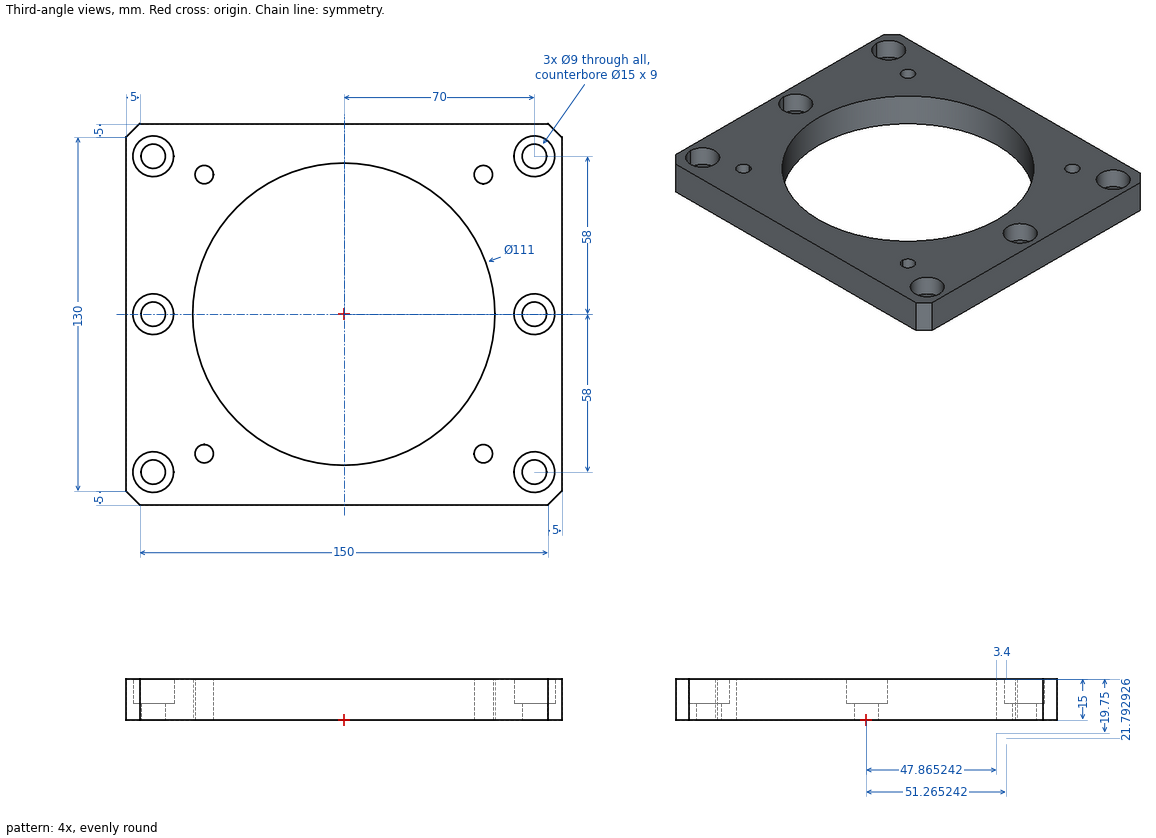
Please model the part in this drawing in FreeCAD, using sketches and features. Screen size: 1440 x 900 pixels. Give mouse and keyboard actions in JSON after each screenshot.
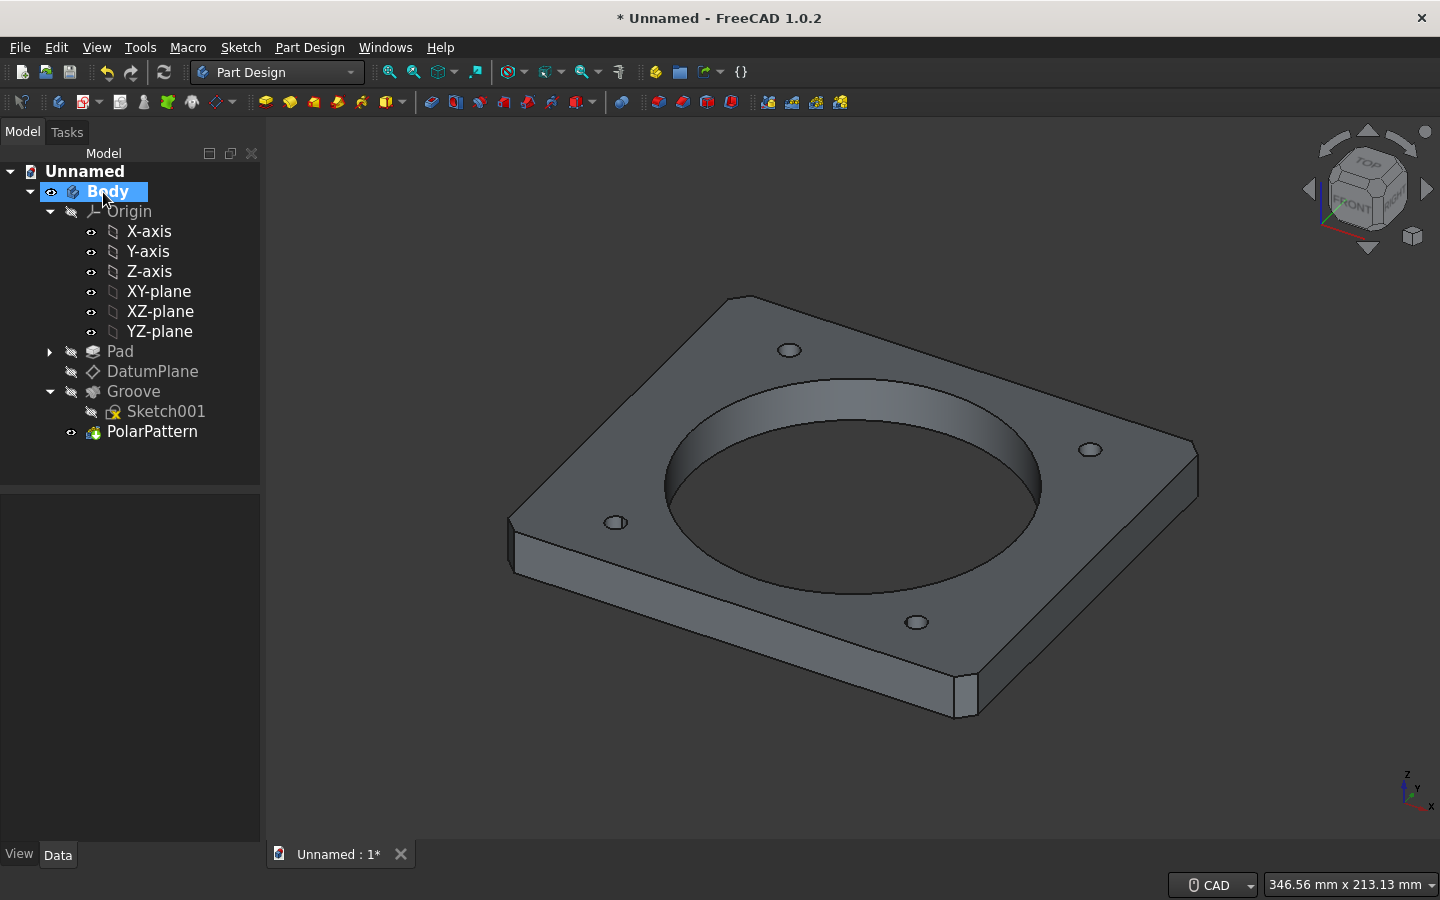
{"action": "left_click", "coordinate": [720, 351]}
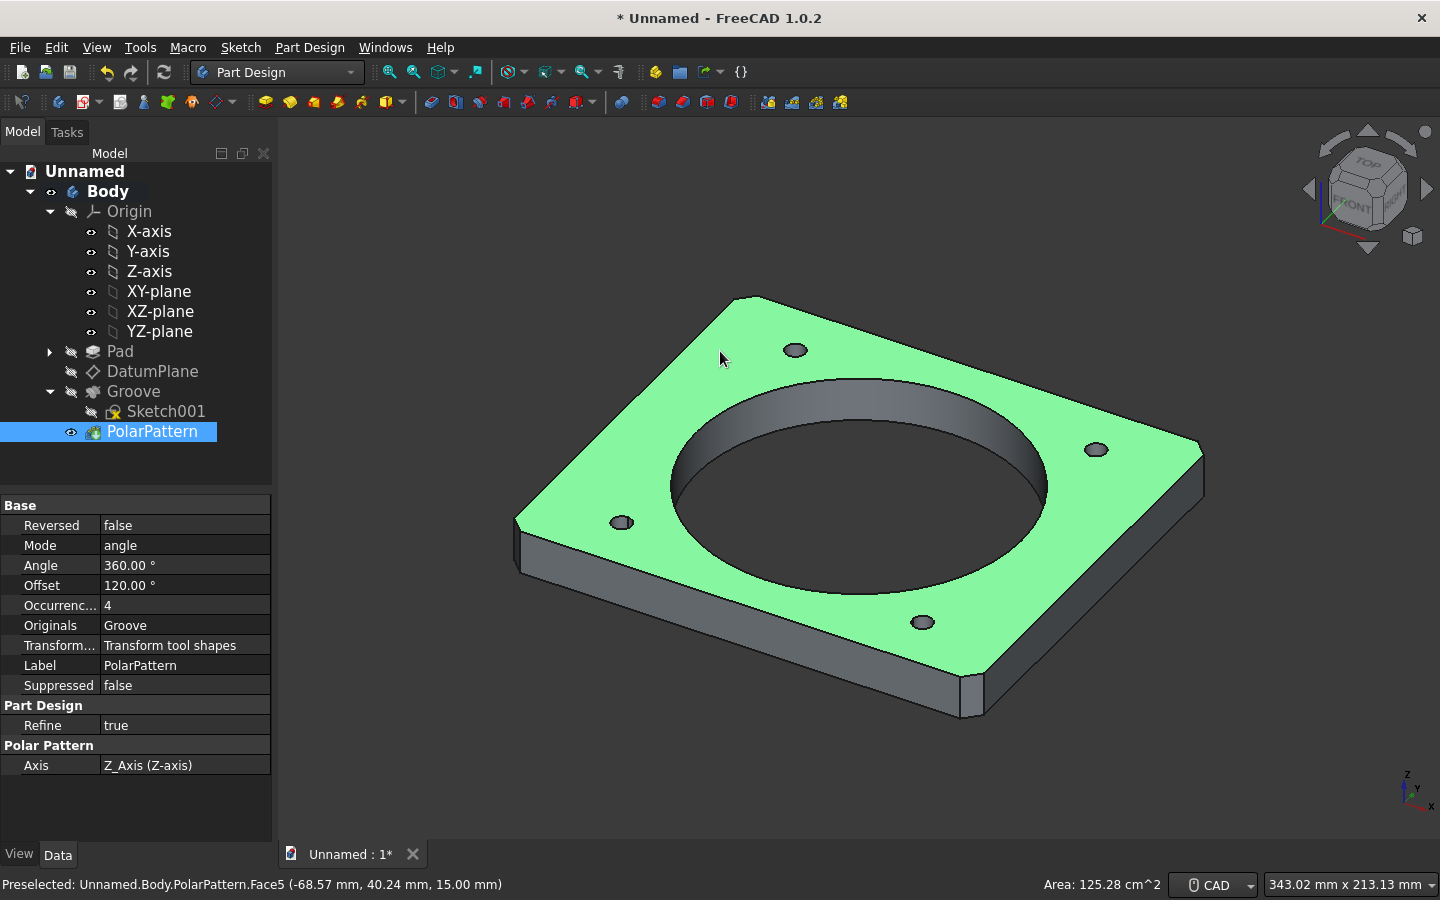
{"action": "left_click", "coordinate": [84, 102]}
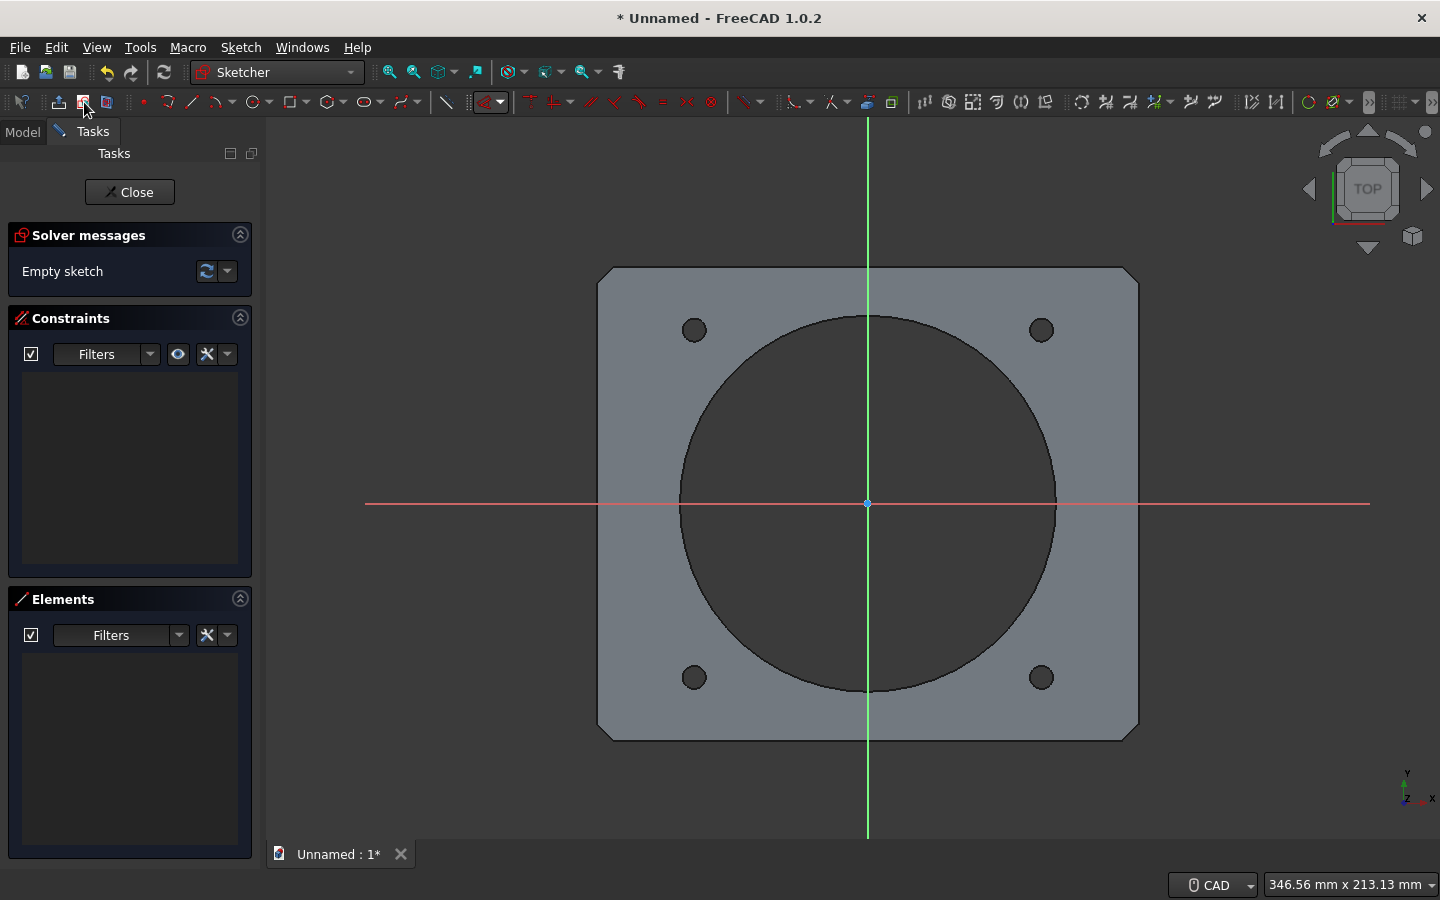
{"action": "left_click", "coordinate": [254, 102]}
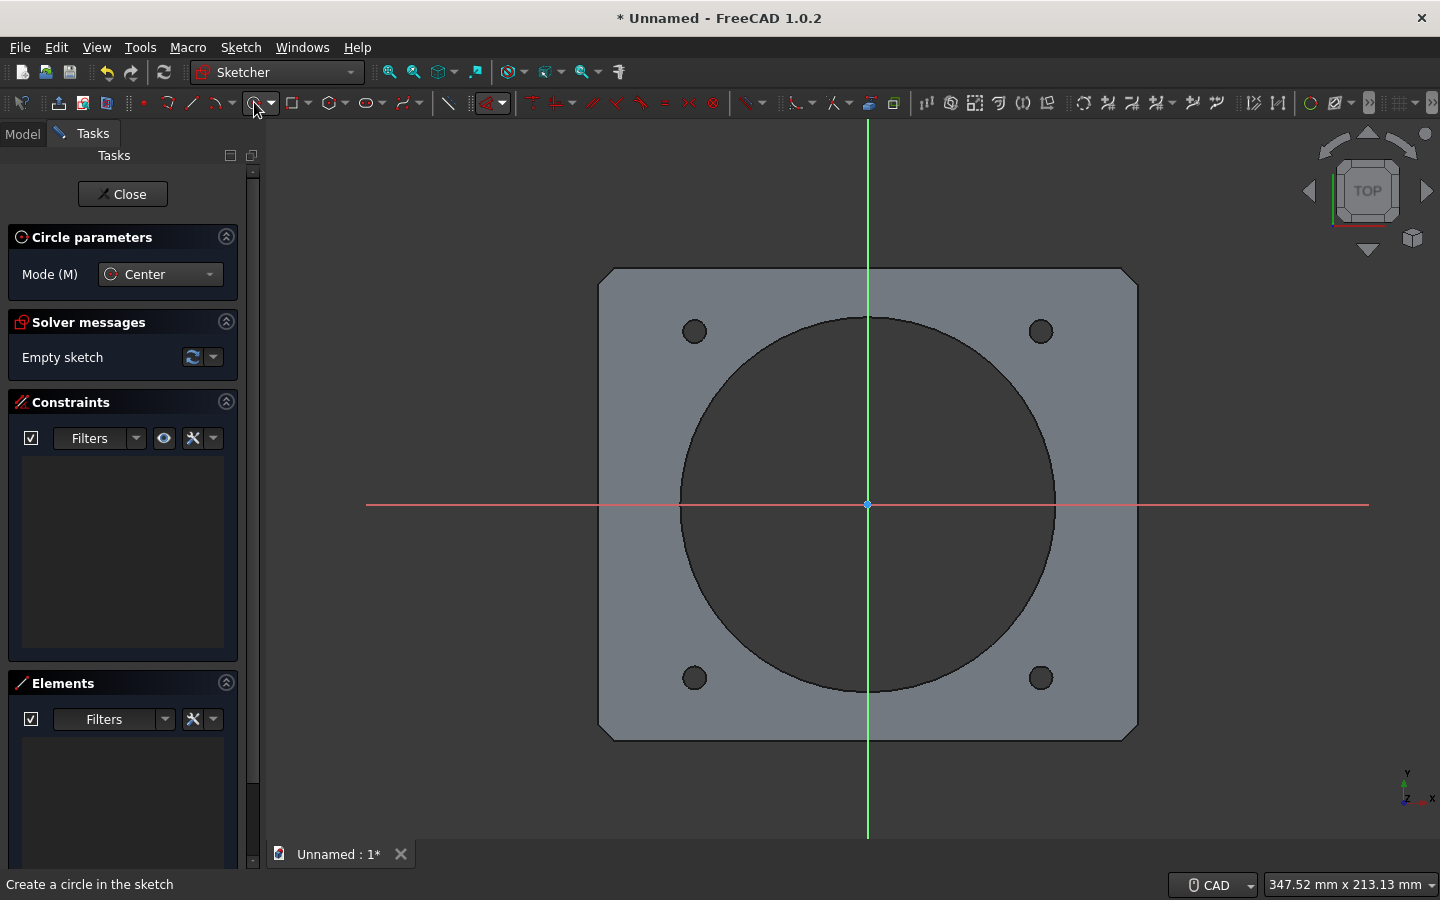
{"action": "scroll", "coordinate": [1104, 309], "scroll_direction": "up", "scroll_amount": 3}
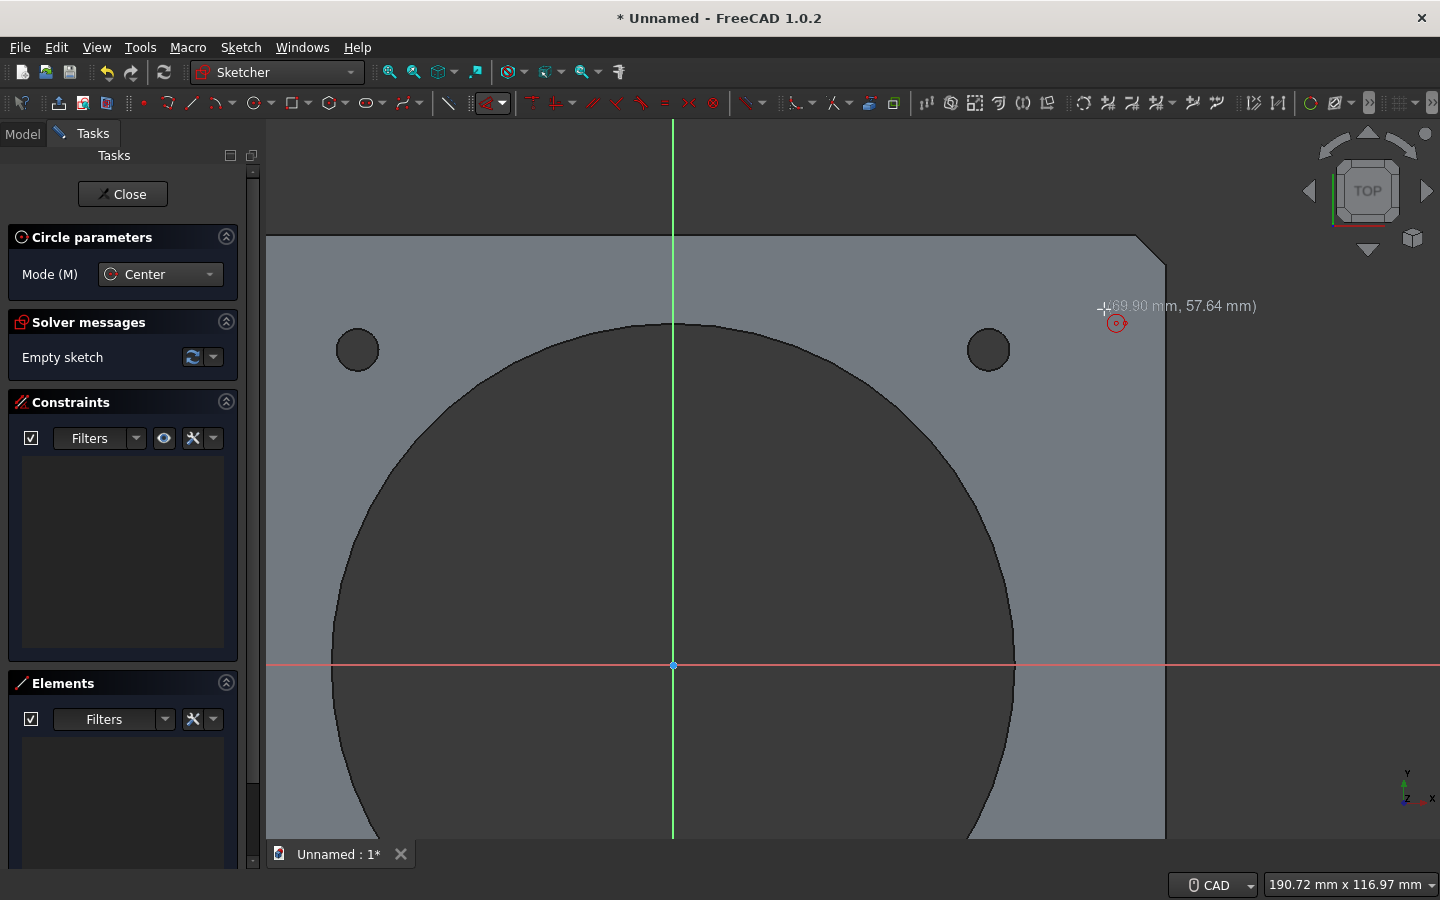
{"action": "left_click", "coordinate": [1104, 308]}
{"action": "mouse_move", "coordinate": [1124, 289]}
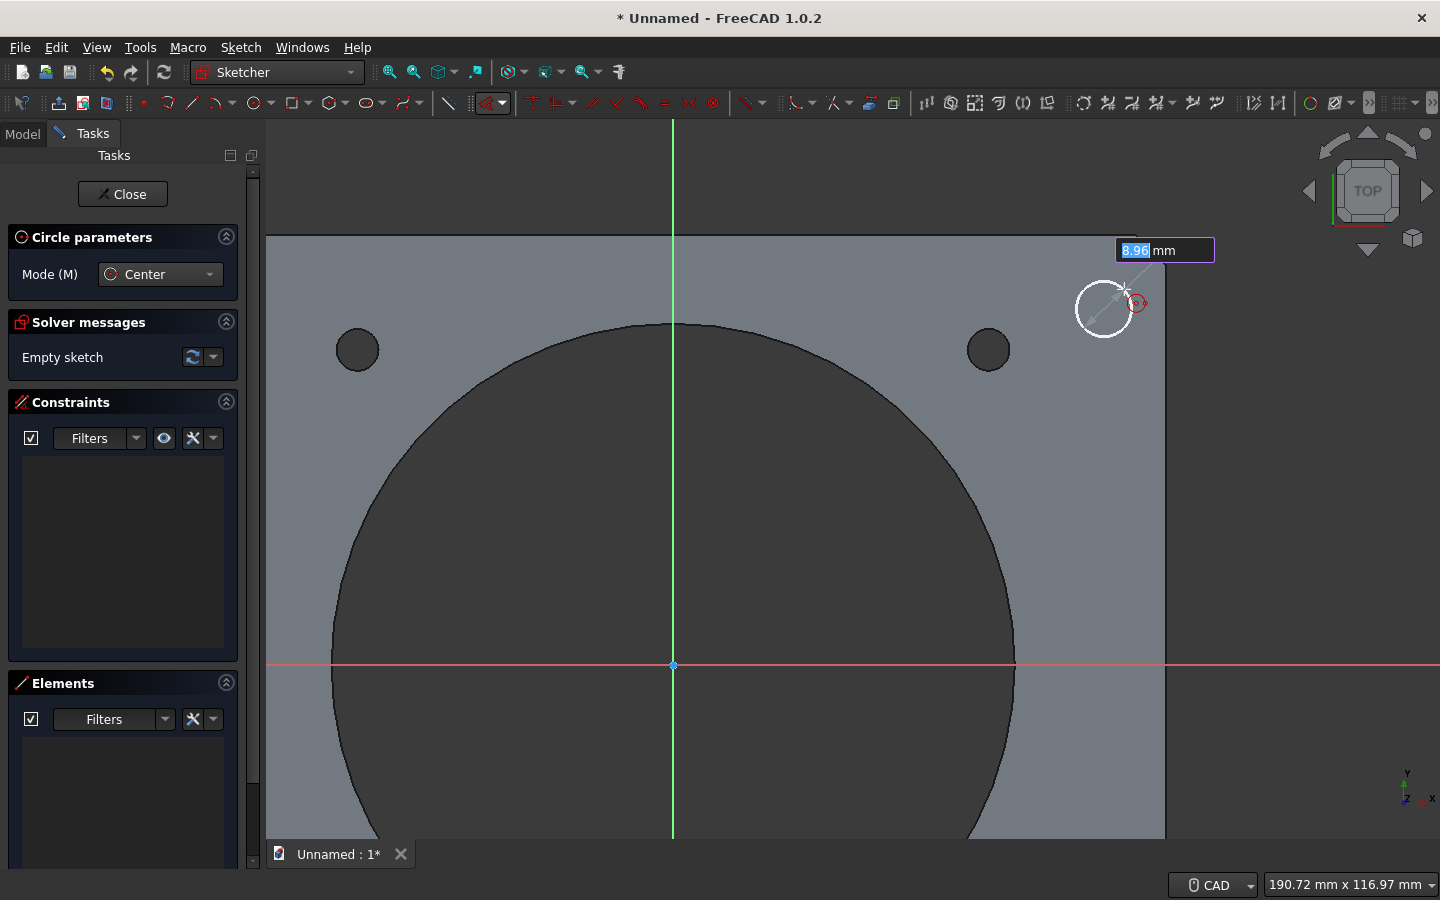
{"action": "type", "text": "9"}
{"action": "key", "text": "Return"}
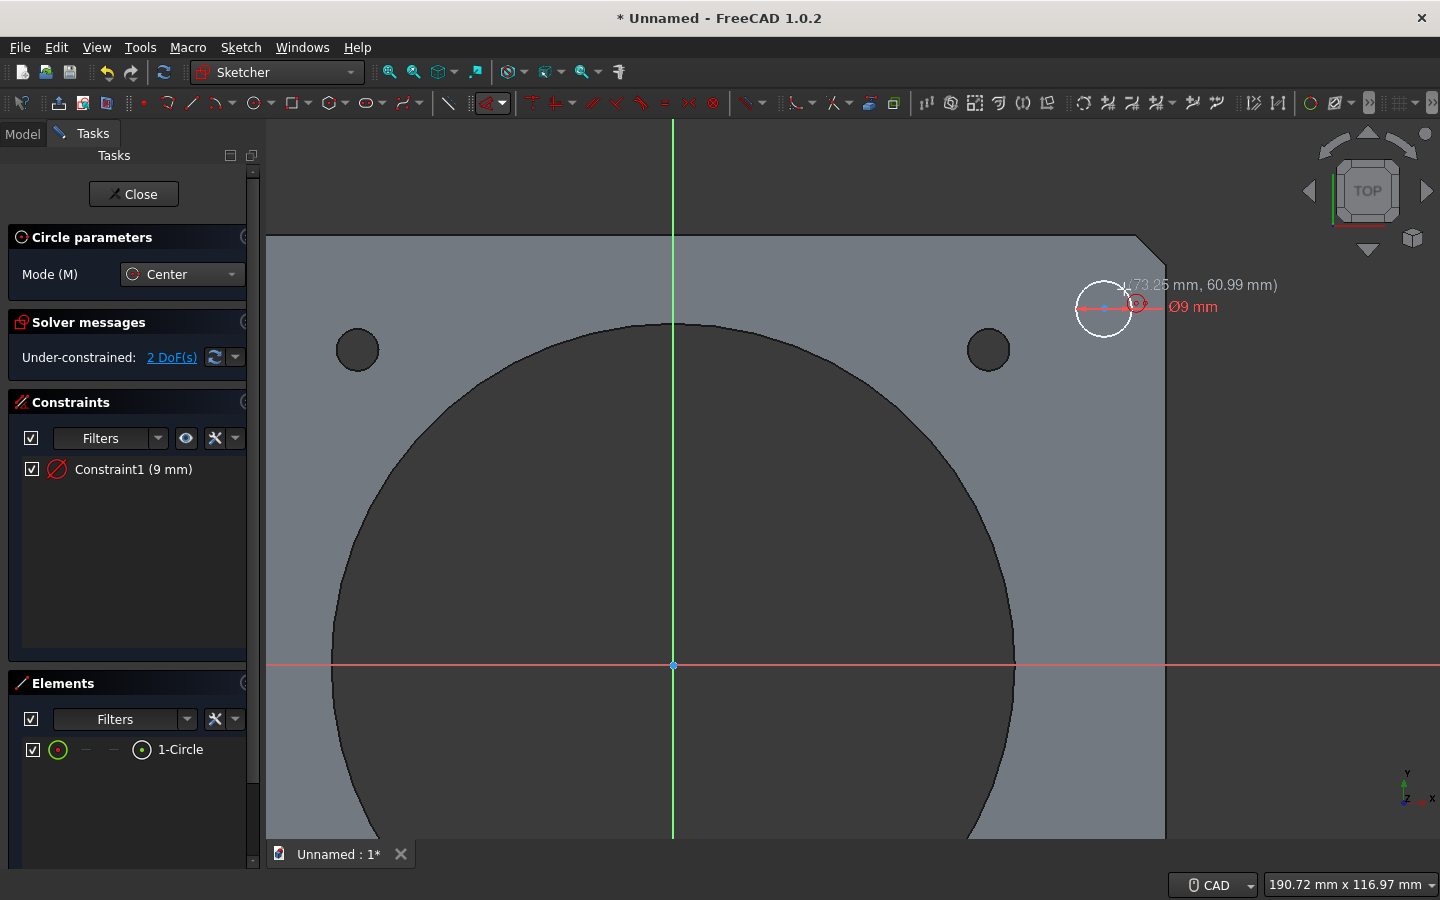
{"action": "left_click", "coordinate": [1104, 665]}
{"action": "mouse_move", "coordinate": [1124, 646]}